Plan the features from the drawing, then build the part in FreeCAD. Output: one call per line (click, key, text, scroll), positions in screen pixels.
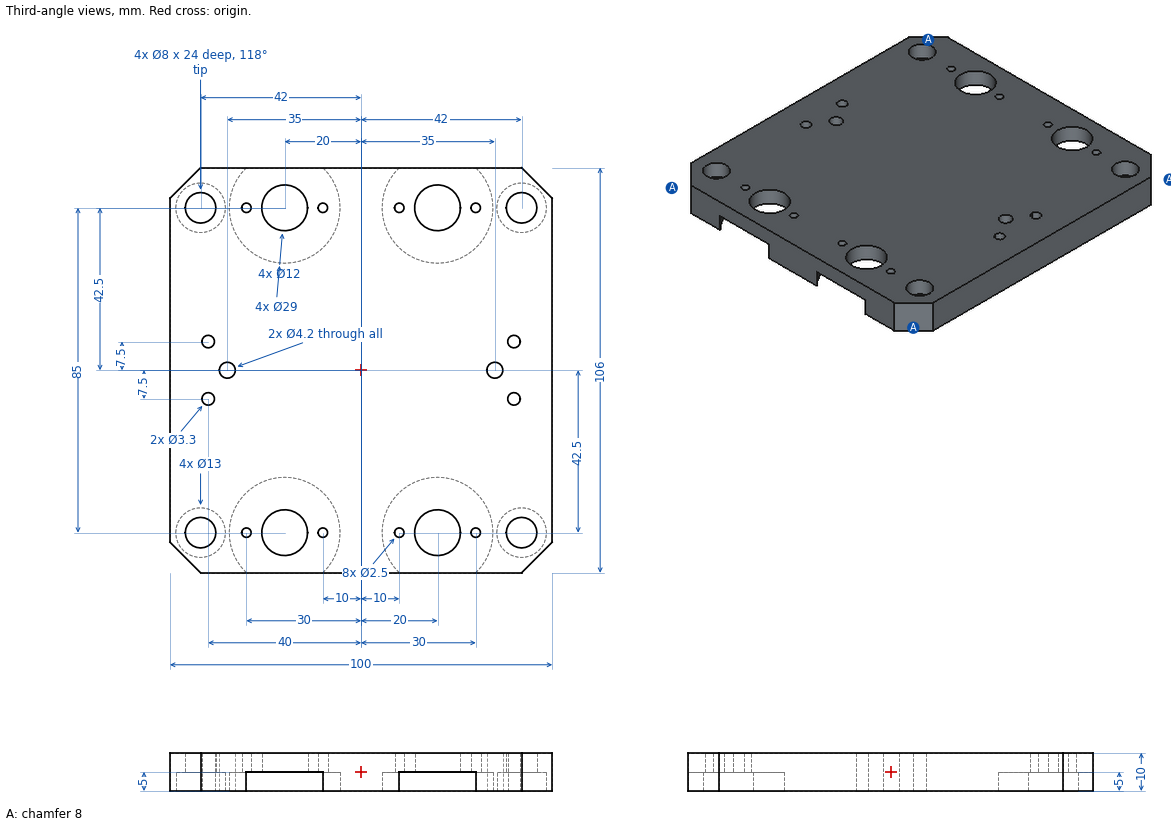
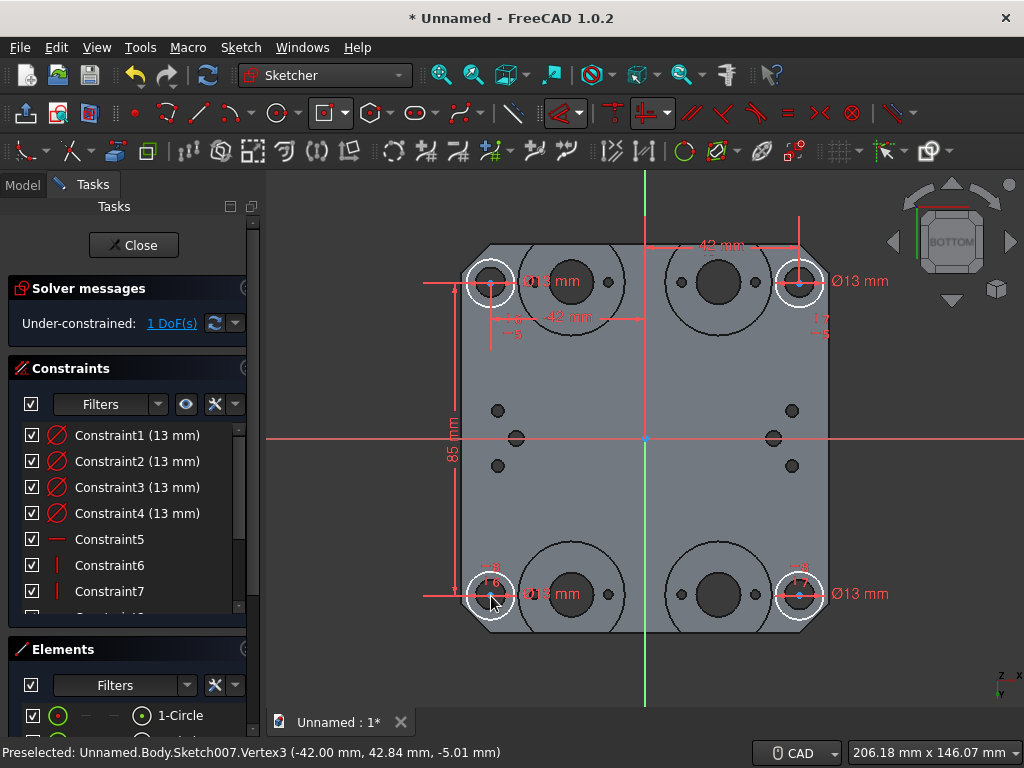
click(491, 283)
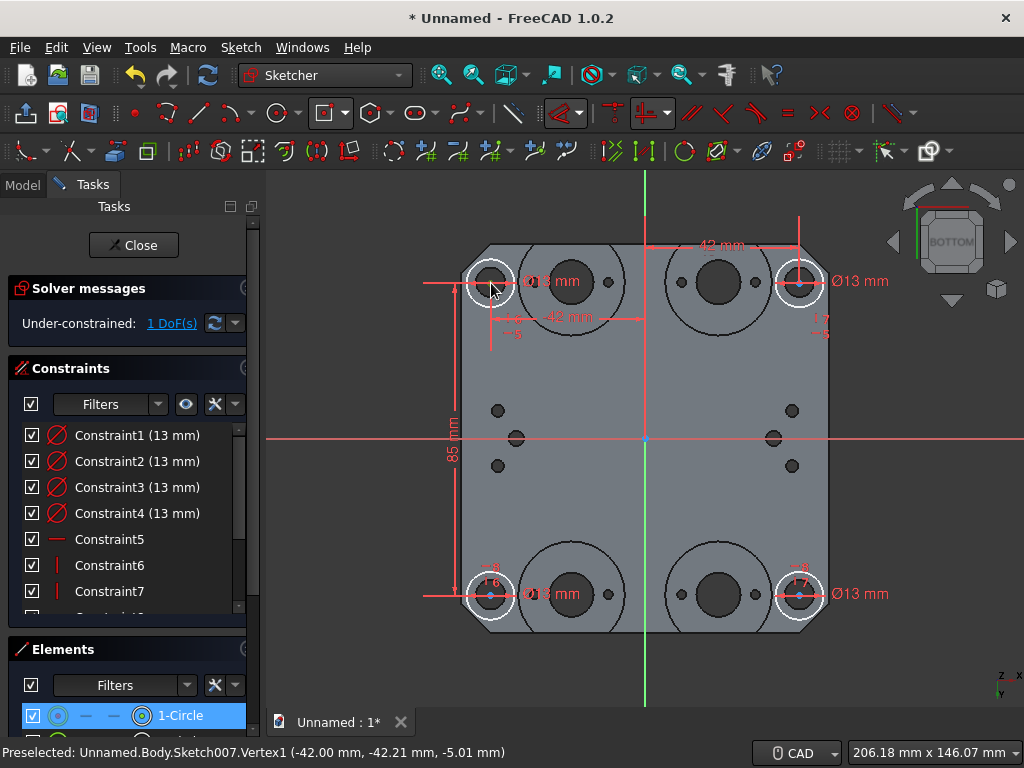
key(i)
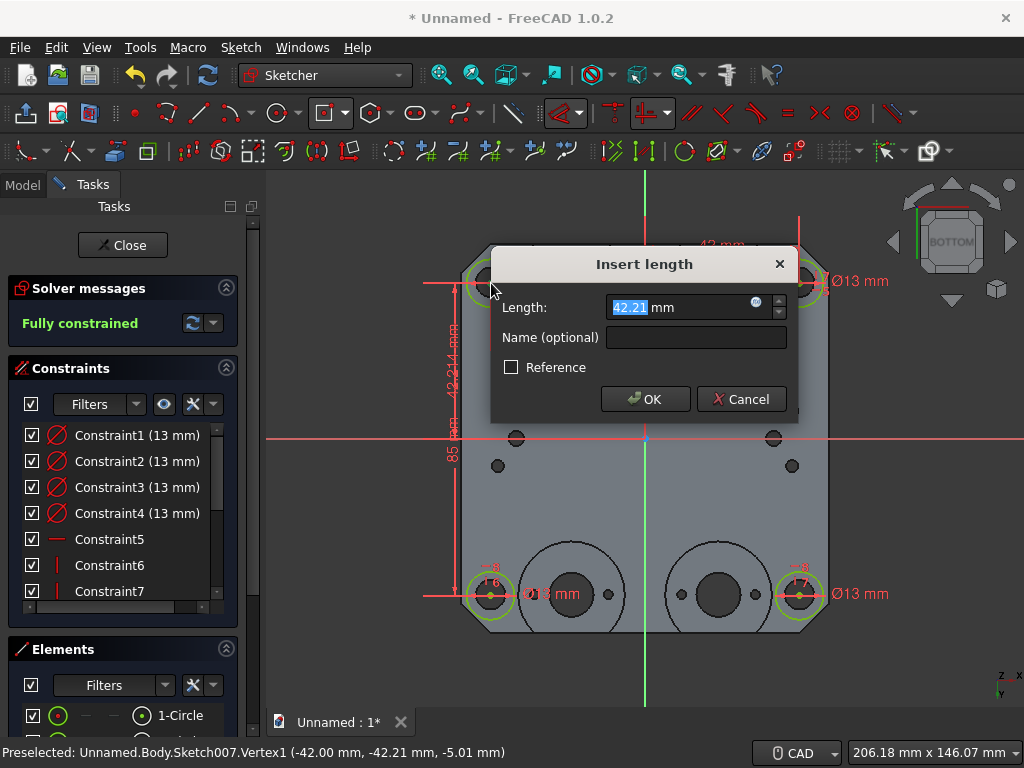
text(42.5)
key(Return)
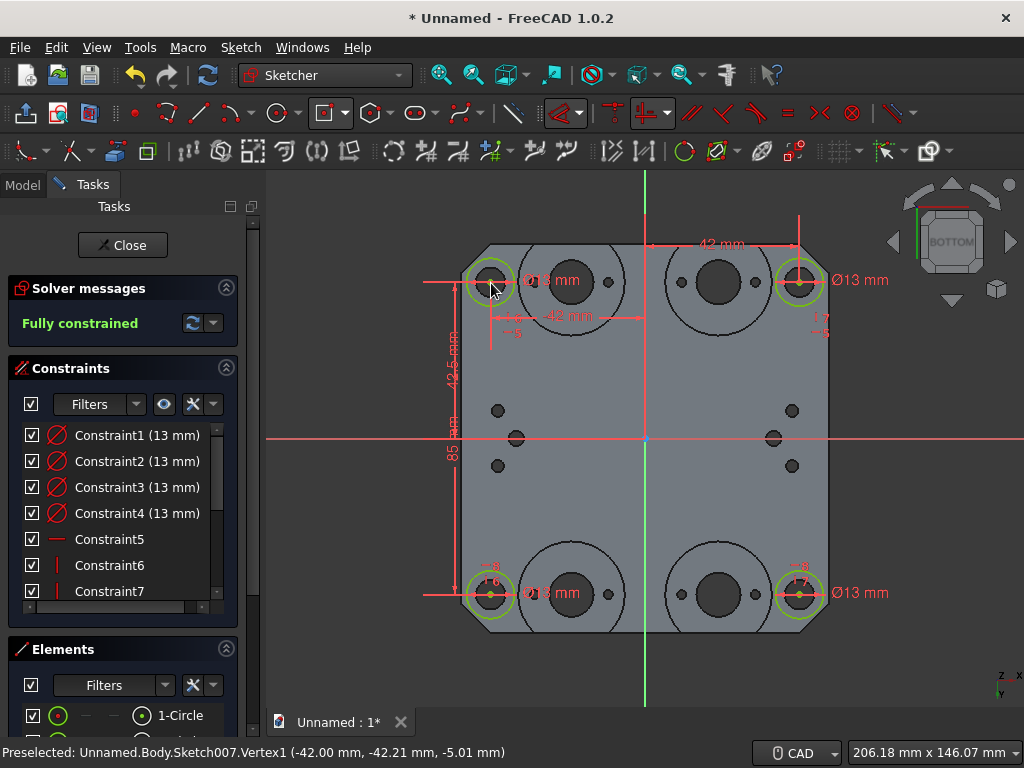
click(123, 245)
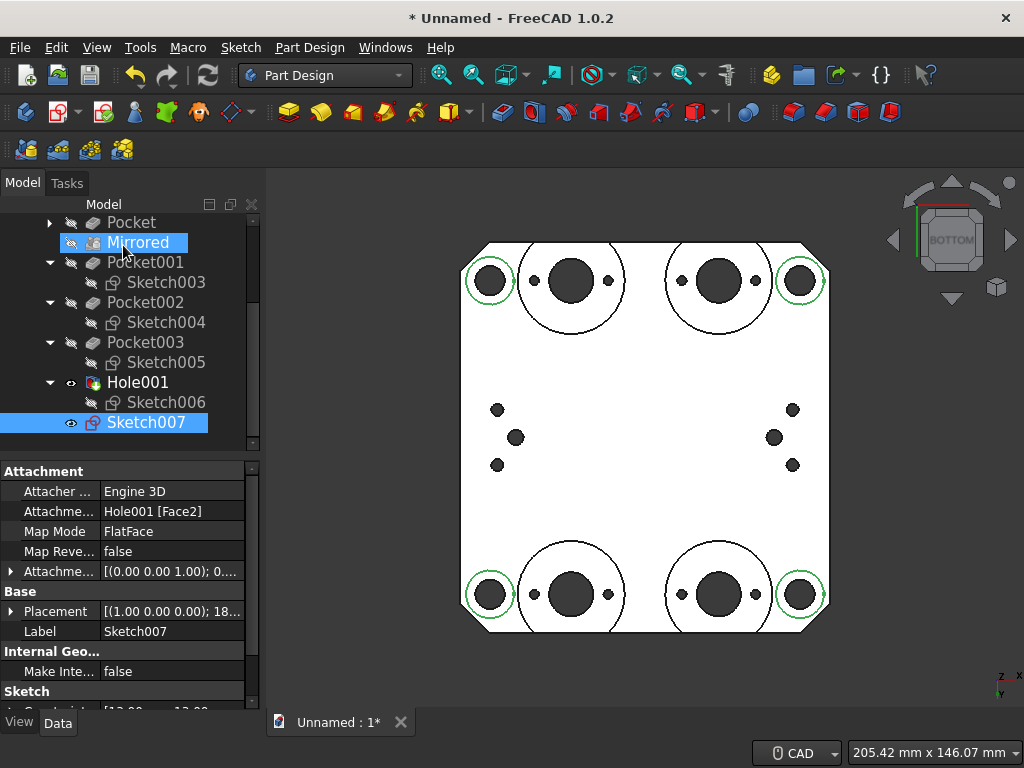
click(504, 112)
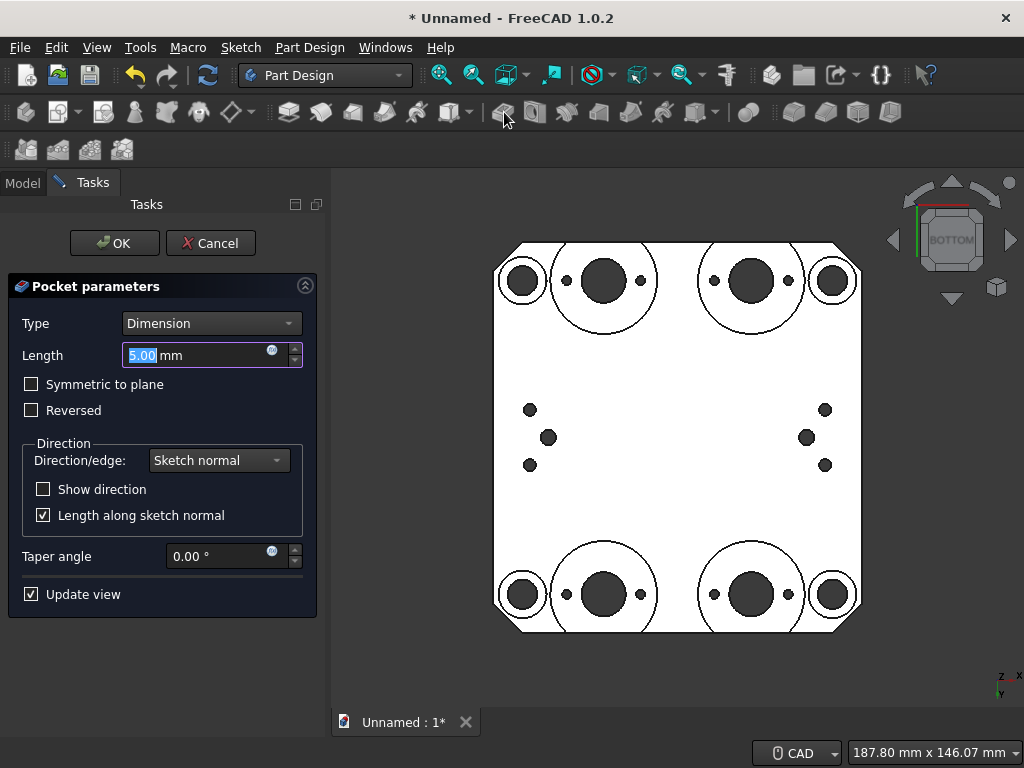
text(5)
key(Tab)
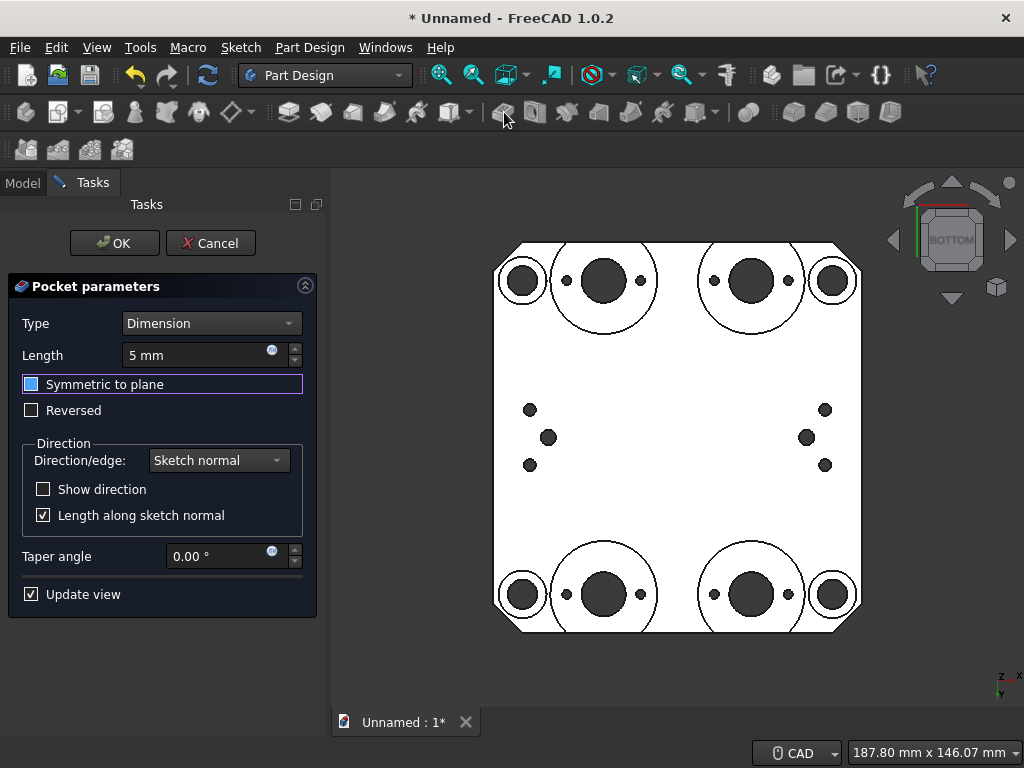
click(115, 243)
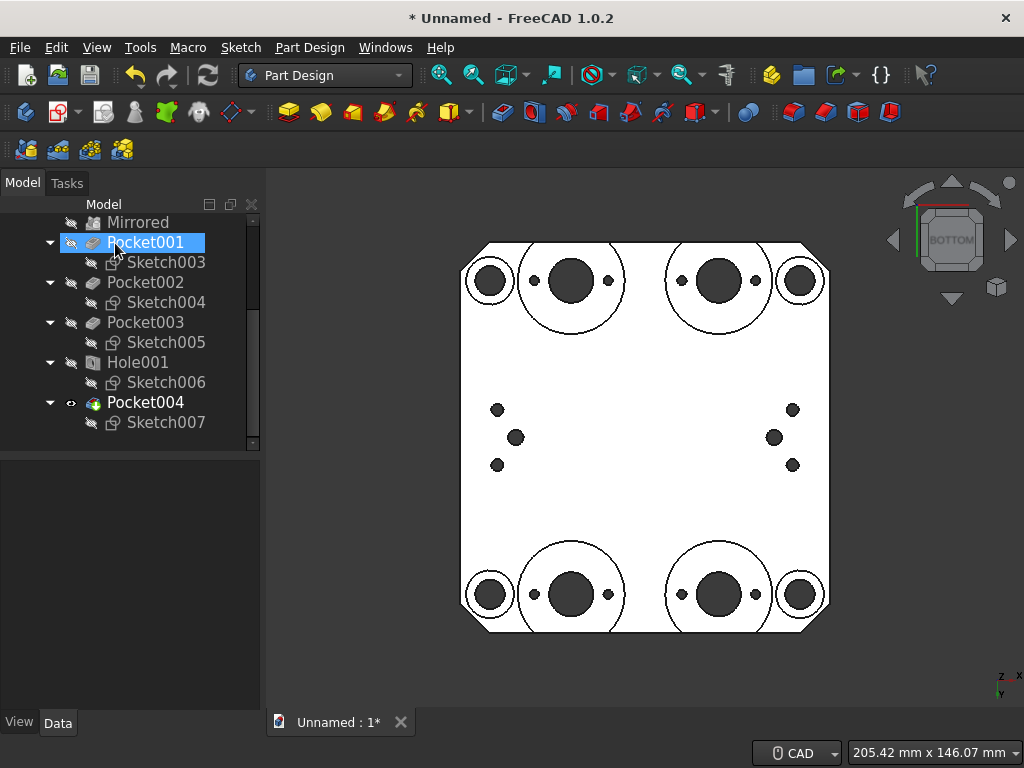
key(0)